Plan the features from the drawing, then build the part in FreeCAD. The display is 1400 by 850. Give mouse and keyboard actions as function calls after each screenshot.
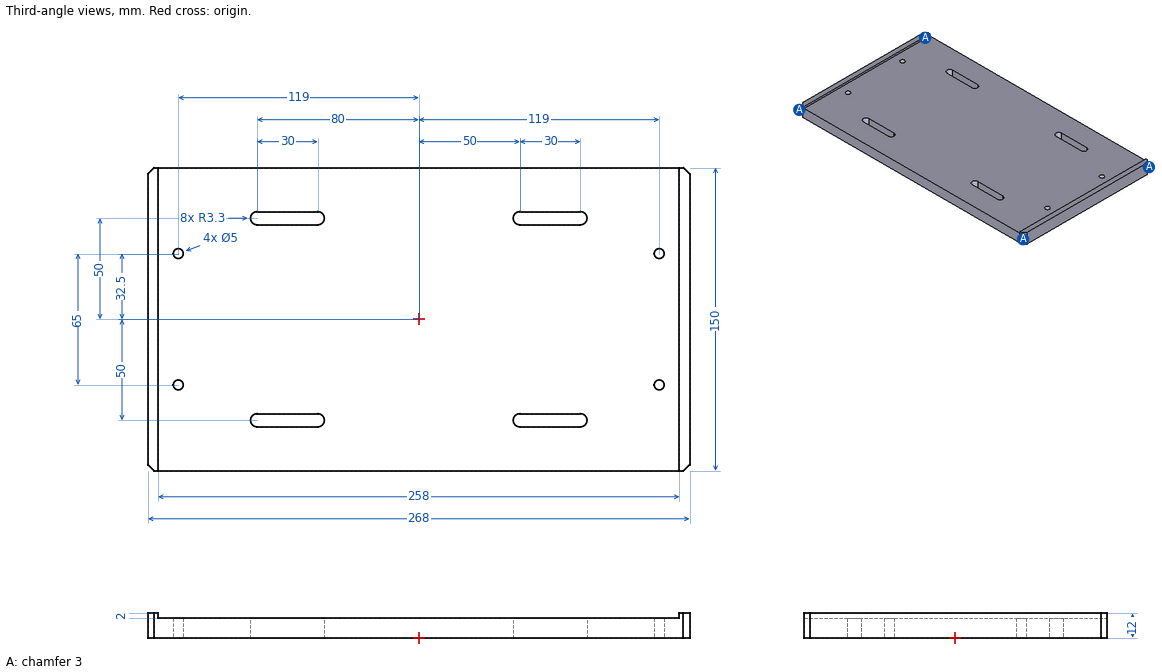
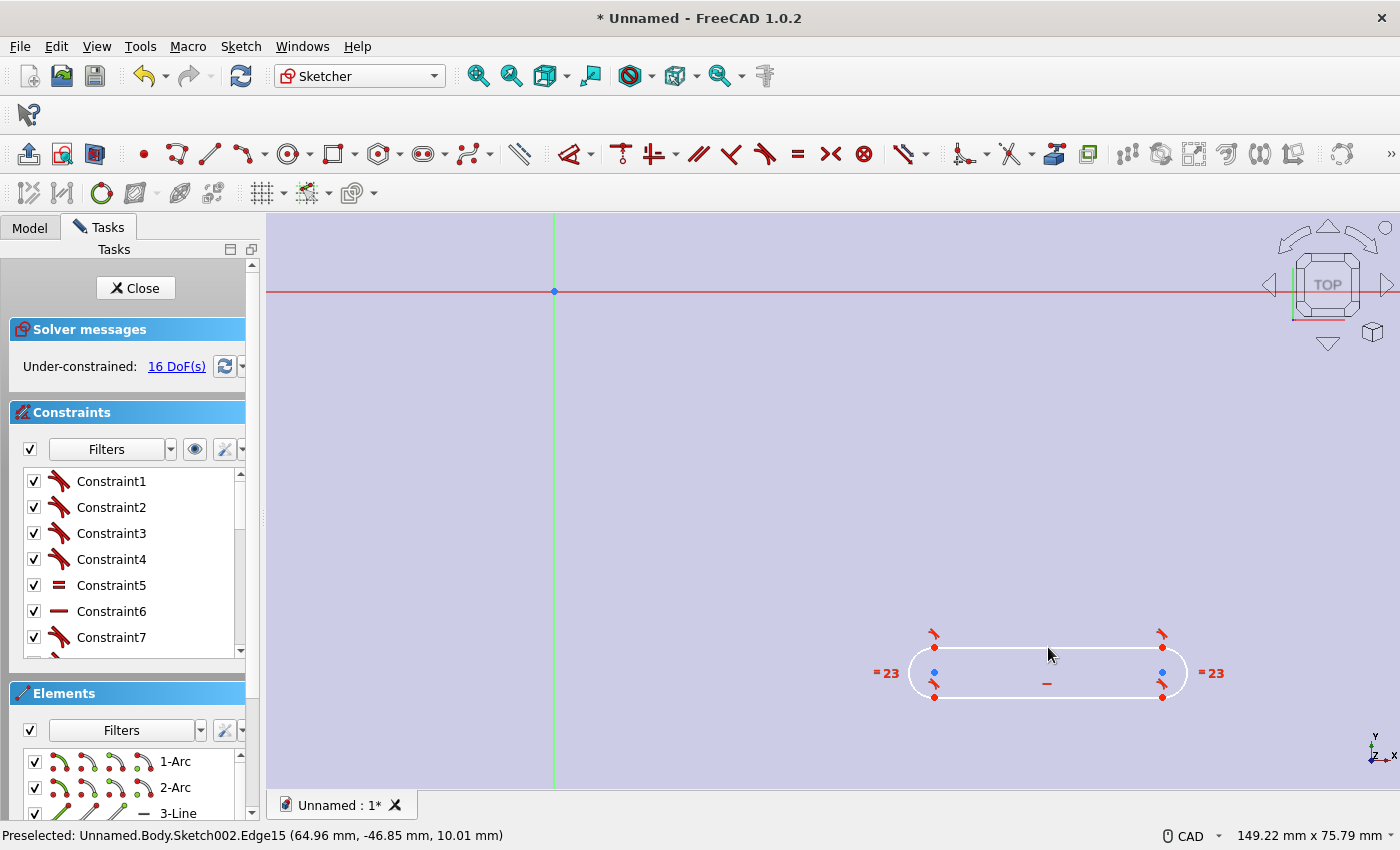
scroll(936, 672, down, 4)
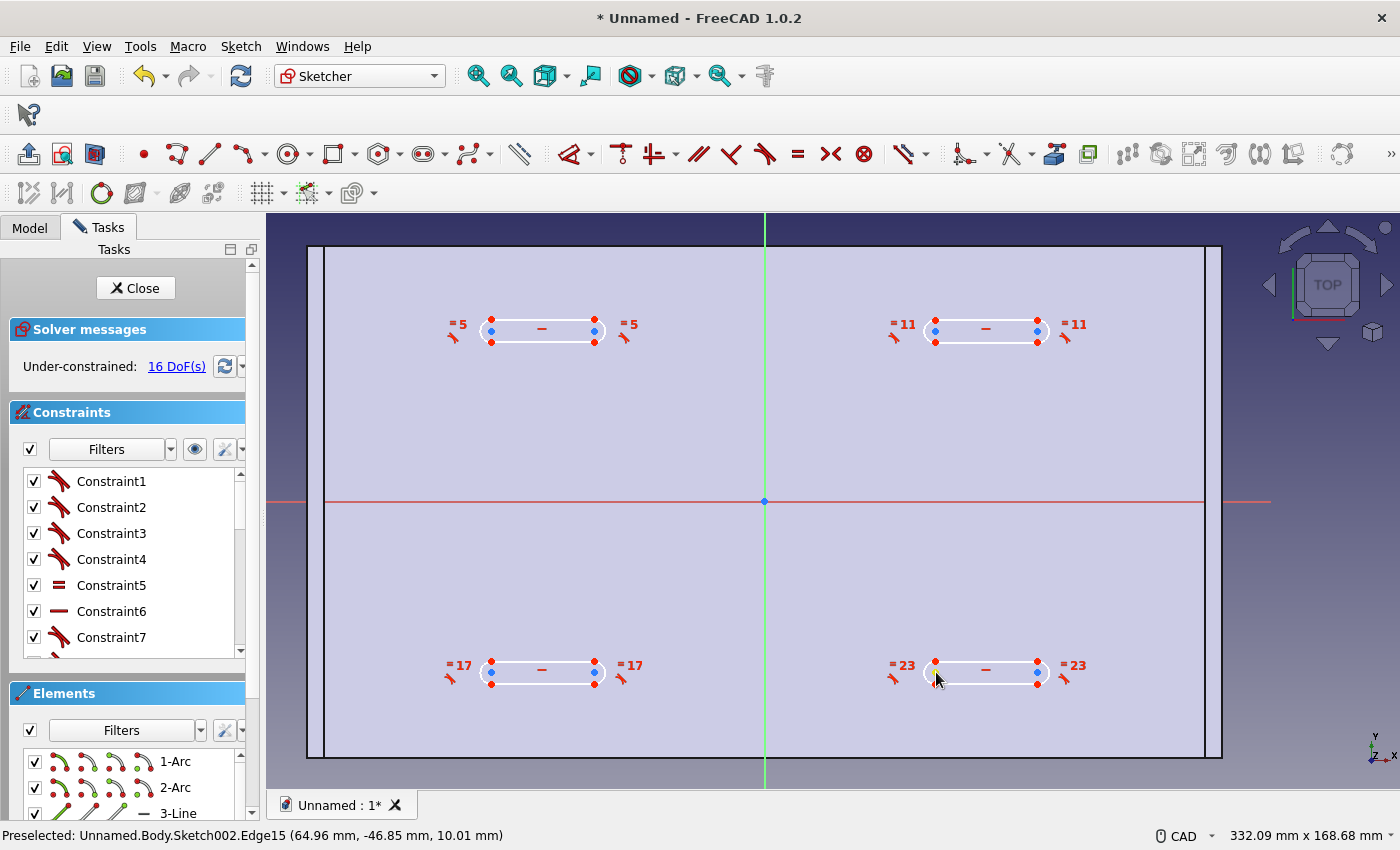
scroll(483, 325, up, 2)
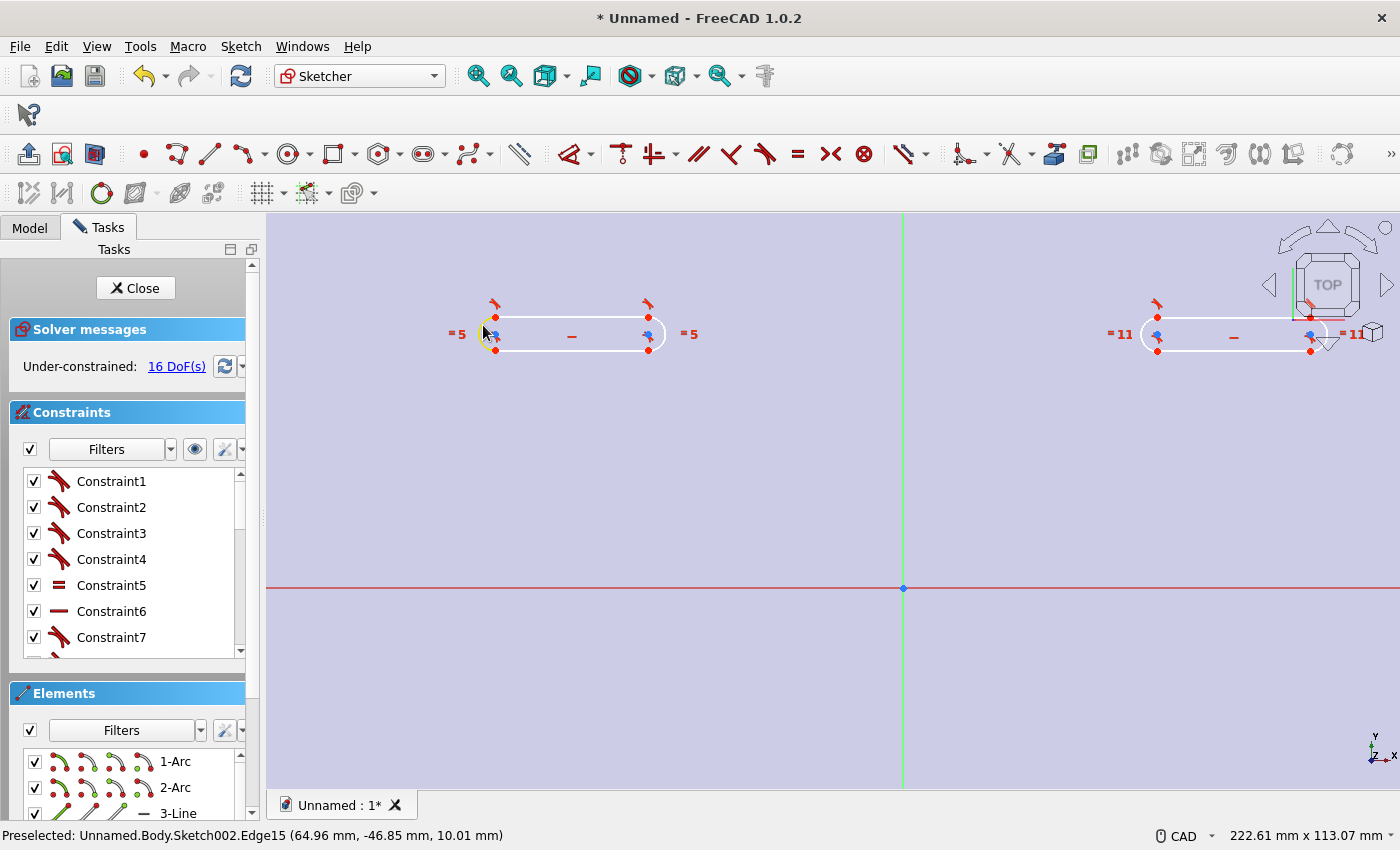
click(482, 324)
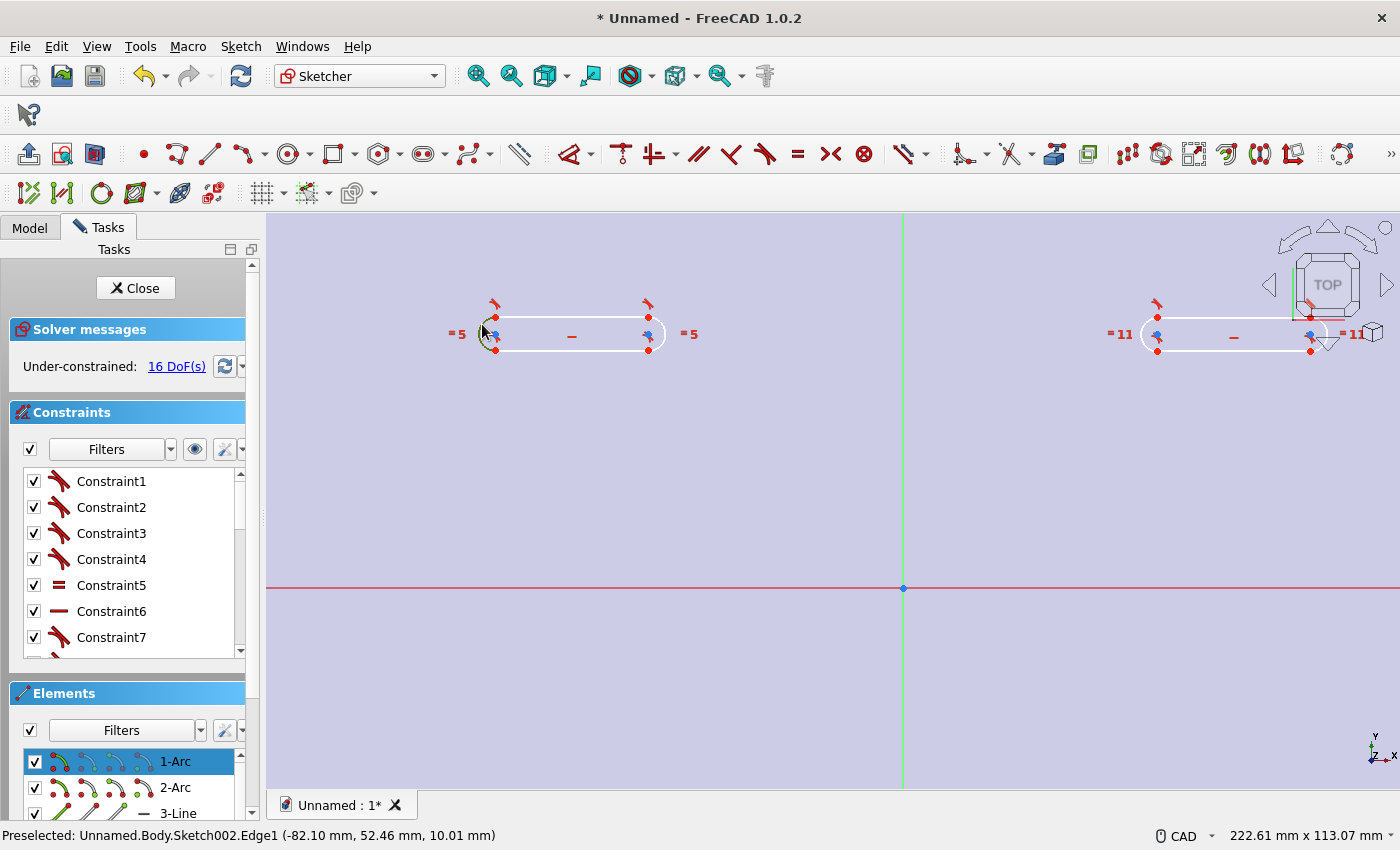
click(1144, 325)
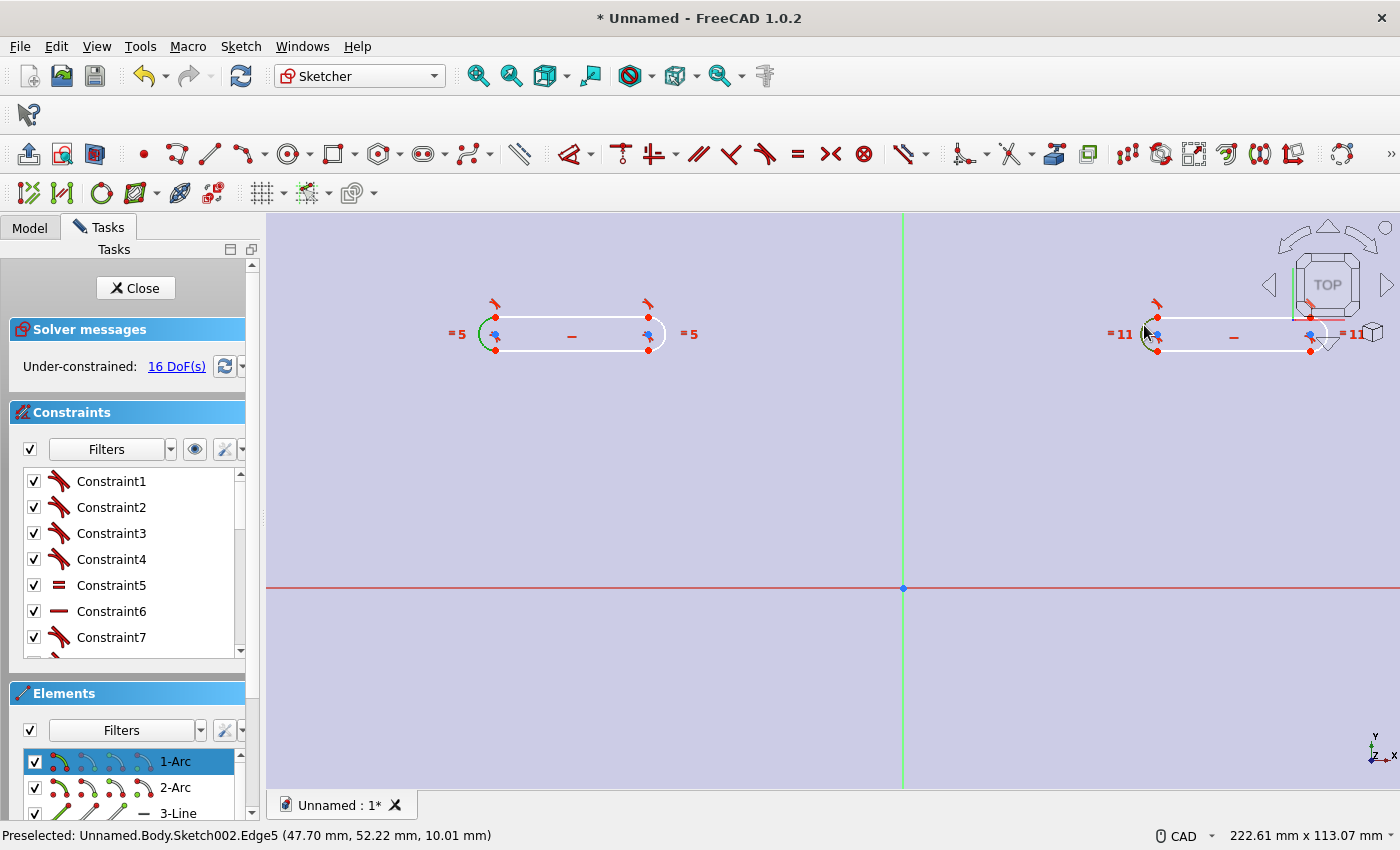
scroll(482, 323, down, 2)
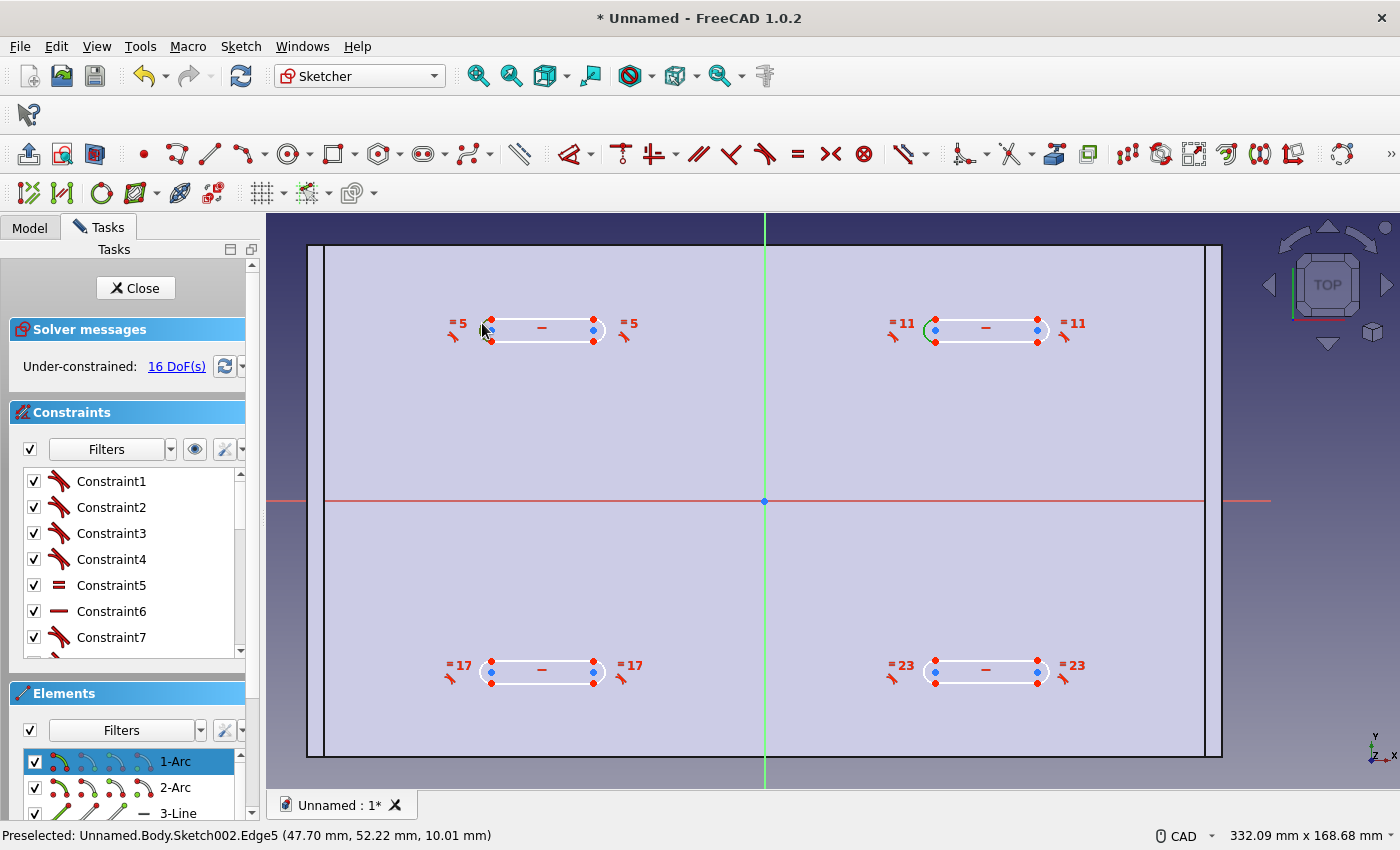
scroll(482, 666, up, 2)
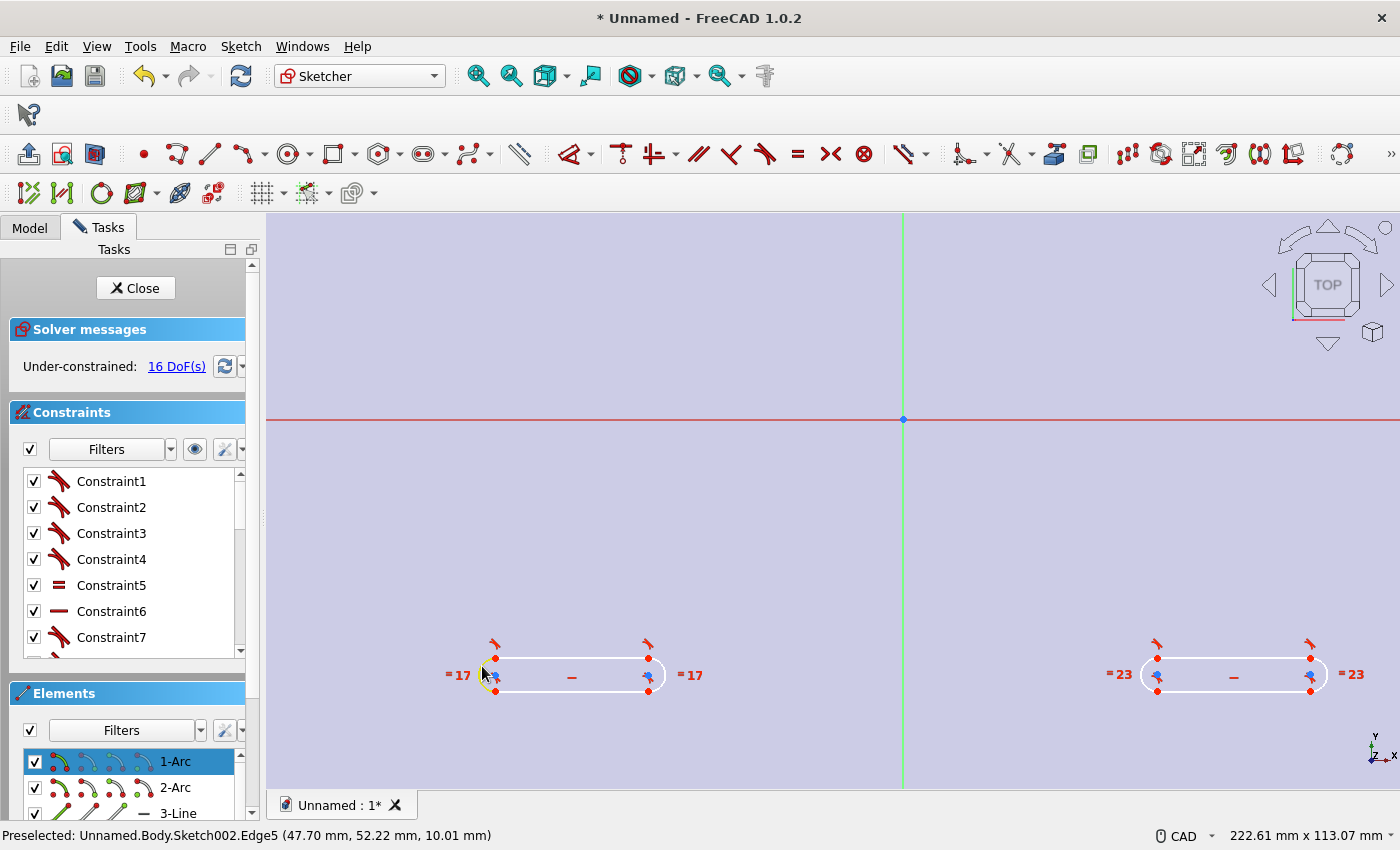
click(482, 665)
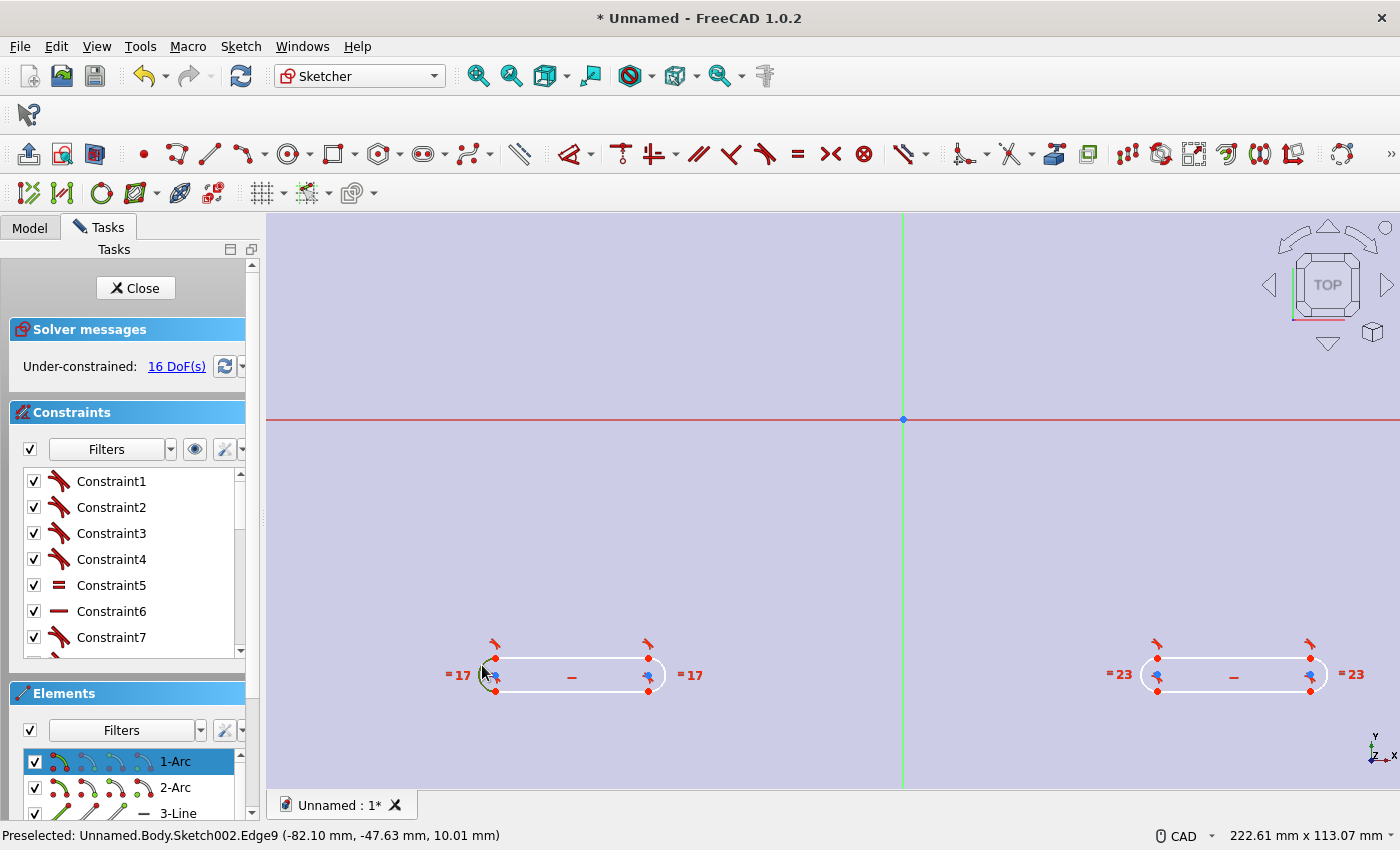
click(1144, 665)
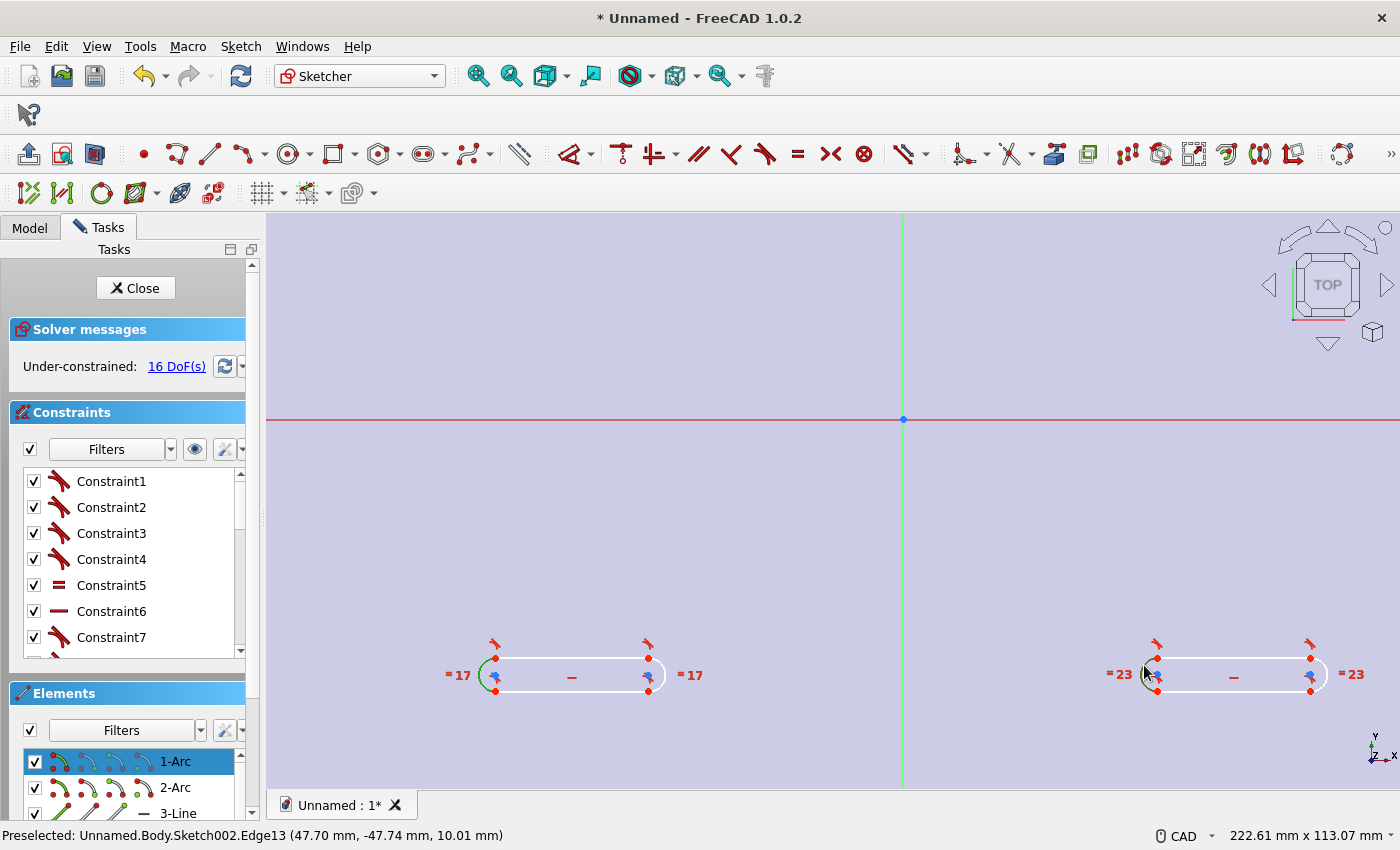
click(798, 154)